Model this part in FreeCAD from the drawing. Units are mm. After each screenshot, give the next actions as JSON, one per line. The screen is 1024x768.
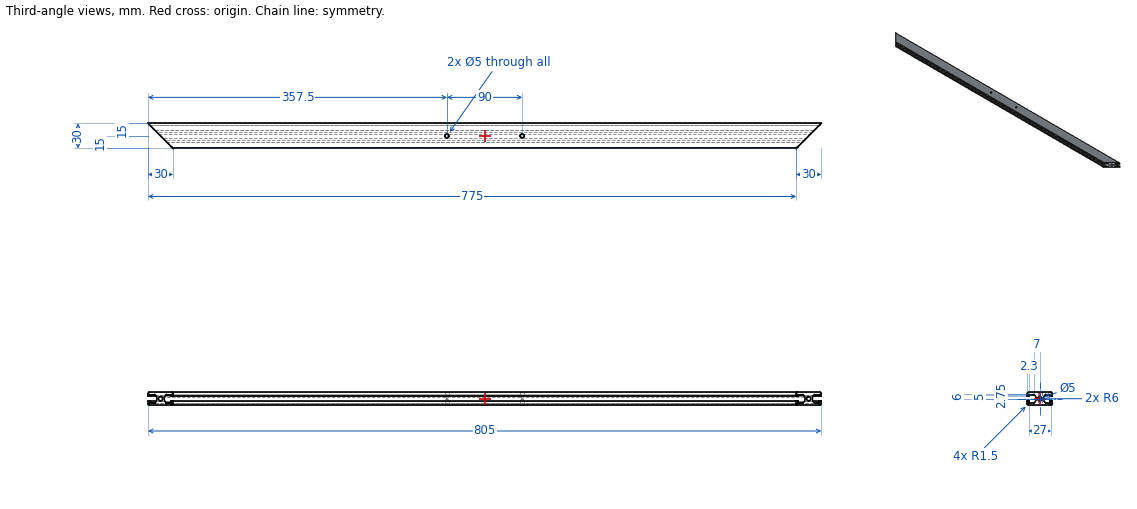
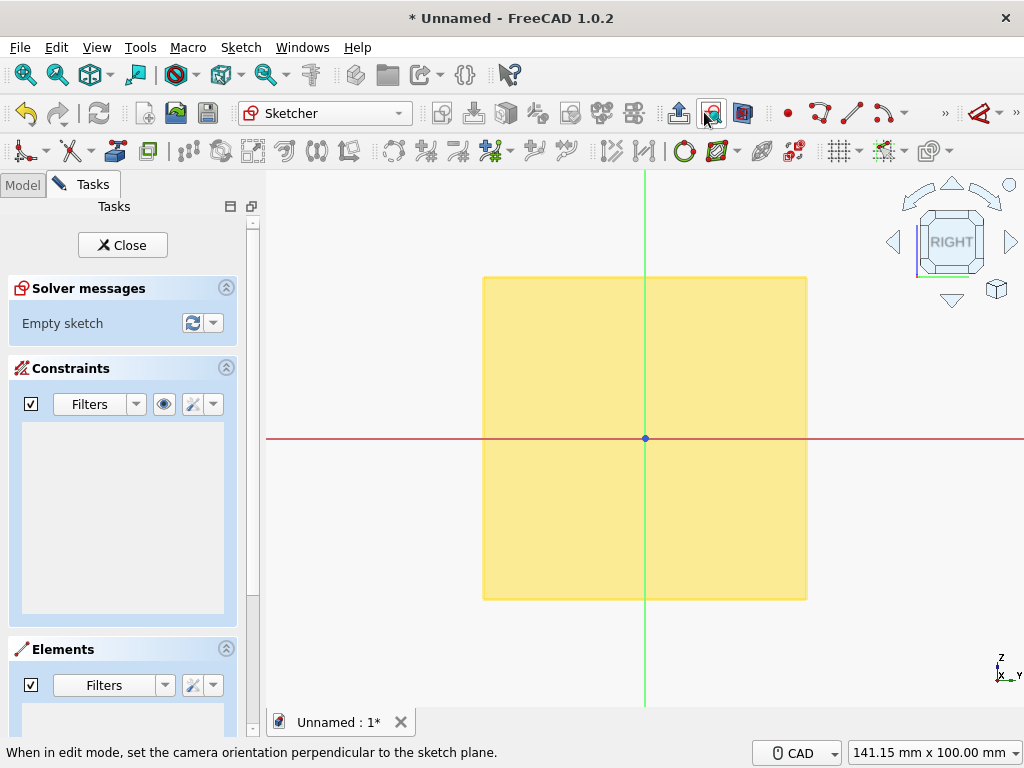
{"action": "scroll", "coordinate": [685, 439], "scroll_direction": "up", "scroll_amount": 5}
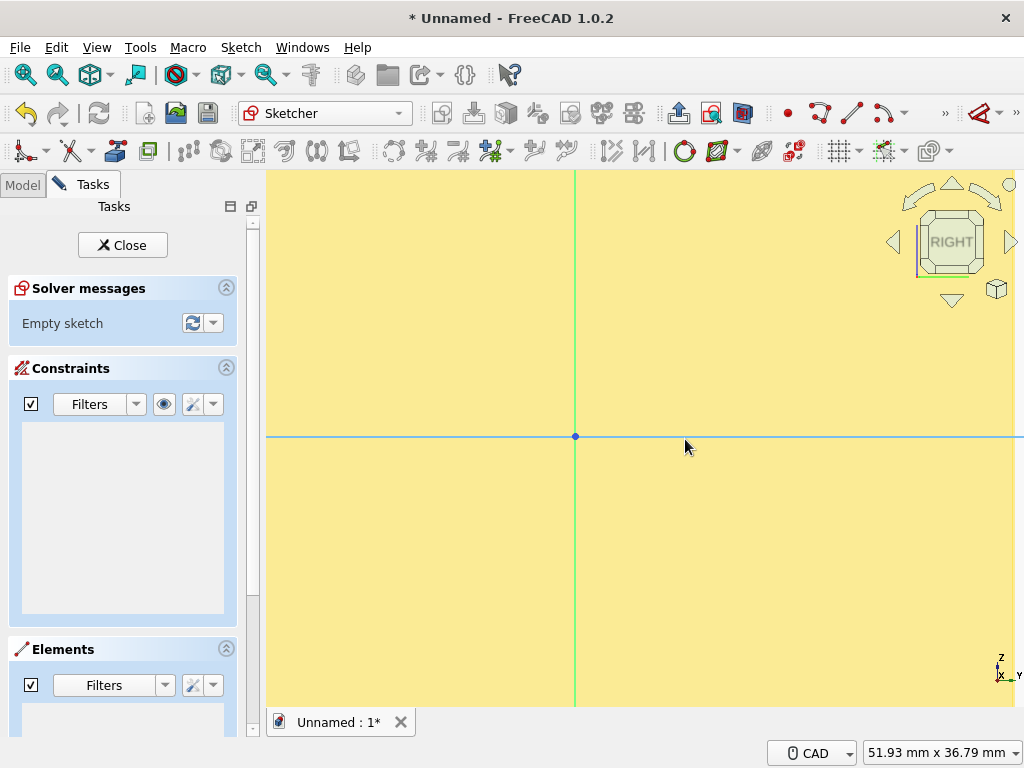
{"action": "left_click", "coordinate": [820, 114]}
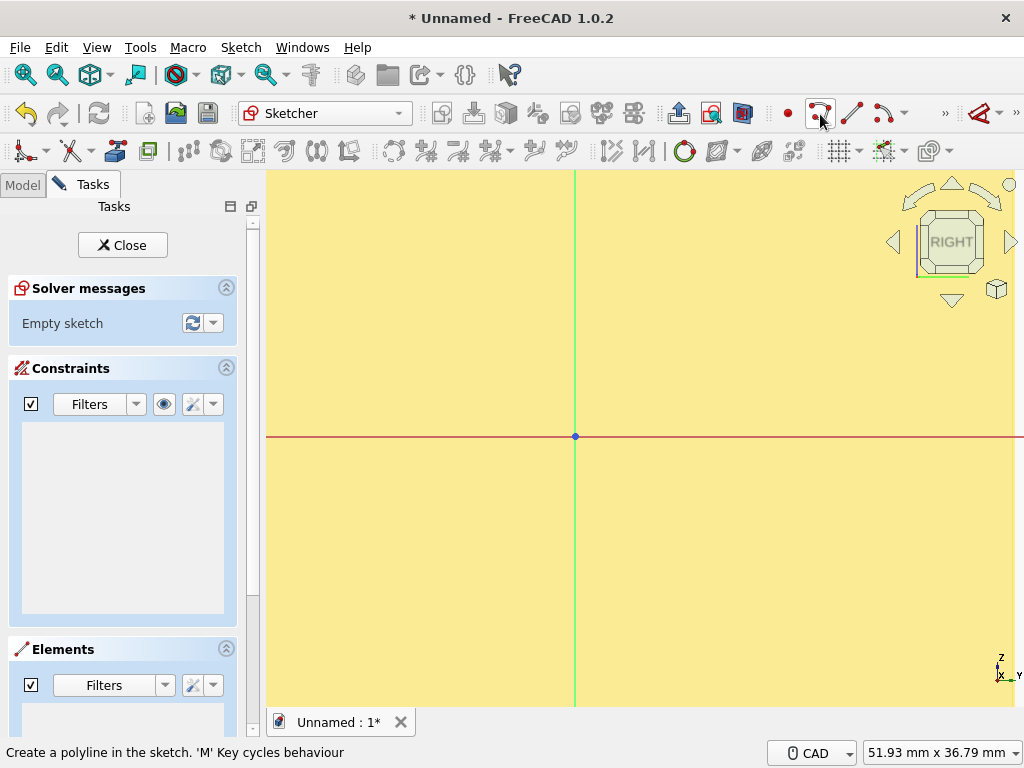
{"action": "left_click", "coordinate": [356, 349]}
{"action": "left_click", "coordinate": [356, 389]}
{"action": "left_click", "coordinate": [390, 389]}
{"action": "left_click", "coordinate": [390, 364]}
{"action": "left_click", "coordinate": [473, 364]}
{"action": "right_click", "coordinate": [473, 364]}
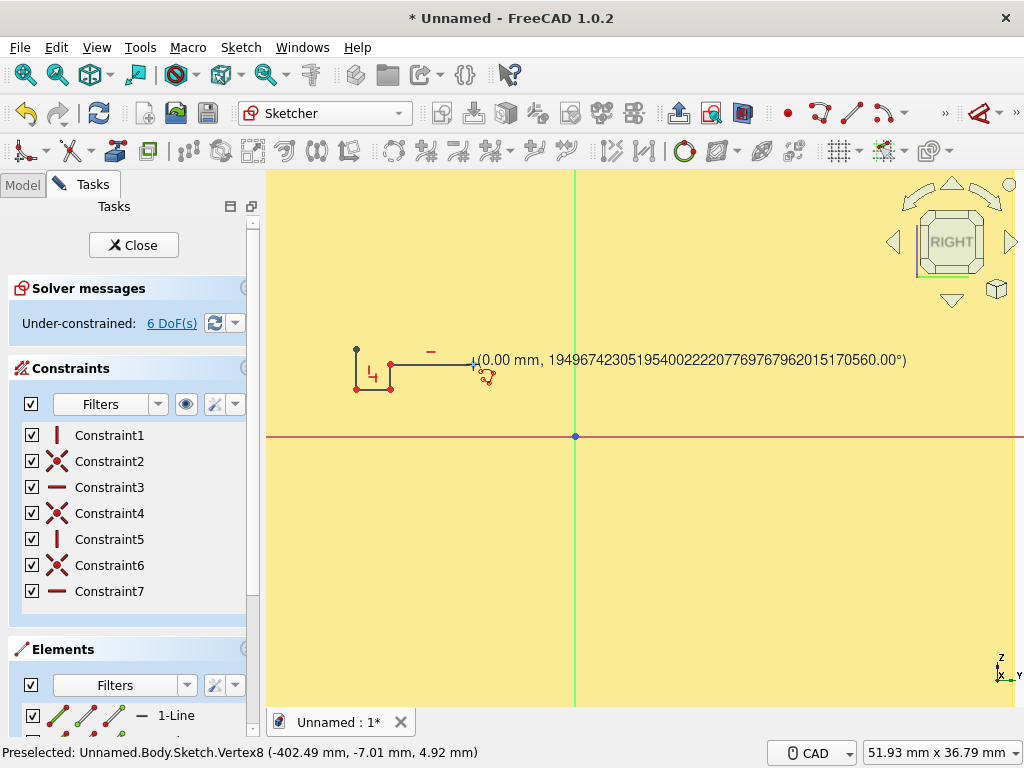
{"action": "left_click", "coordinate": [473, 510]}
{"action": "left_click", "coordinate": [390, 510]}
{"action": "left_click", "coordinate": [390, 484]}
{"action": "left_click", "coordinate": [356, 484]}
{"action": "left_click", "coordinate": [356, 524]}
{"action": "right_click", "coordinate": [356, 524]}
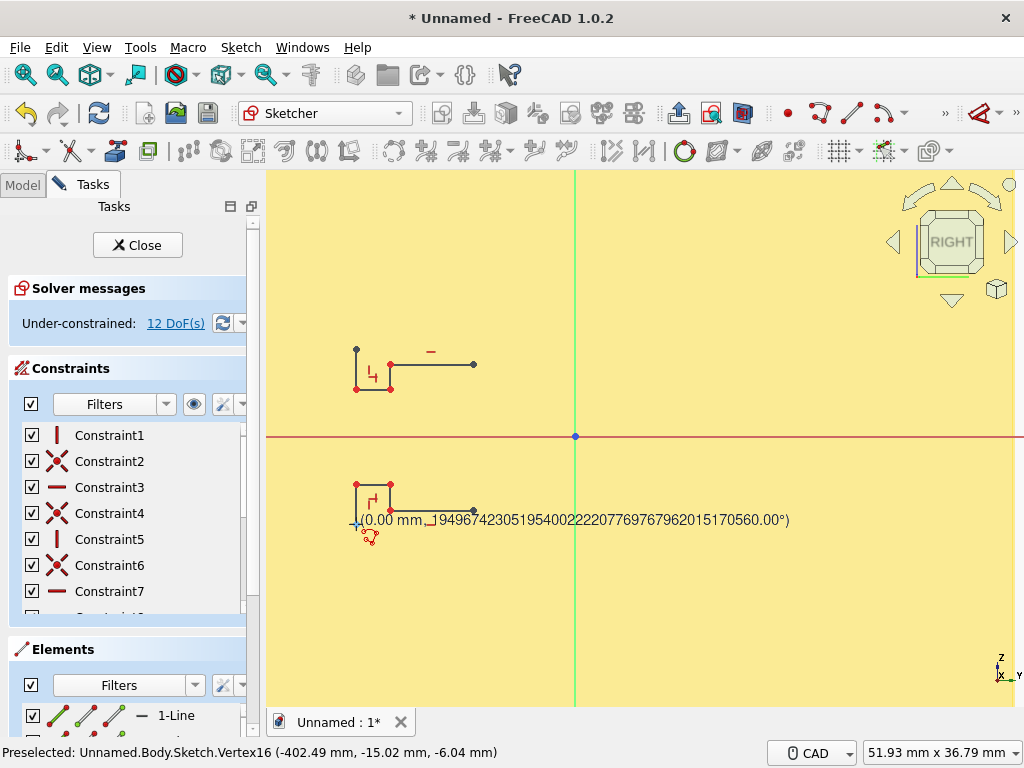
{"action": "left_click", "coordinate": [852, 114]}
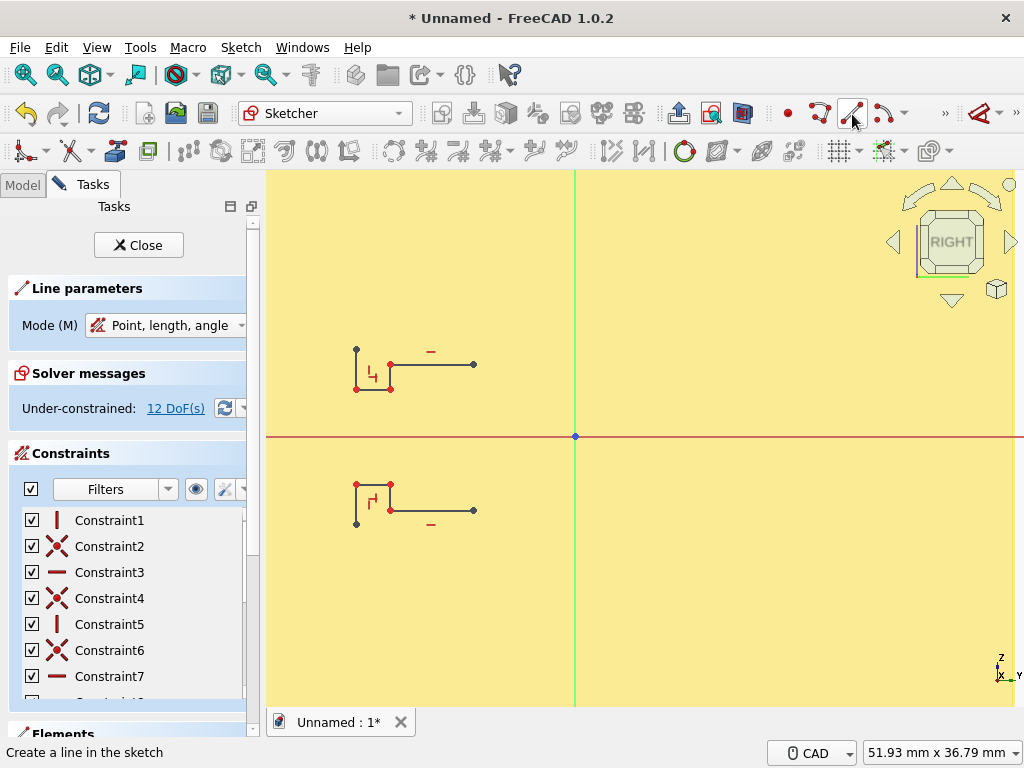
{"action": "left_click", "coordinate": [378, 546]}
{"action": "left_click", "coordinate": [772, 546]}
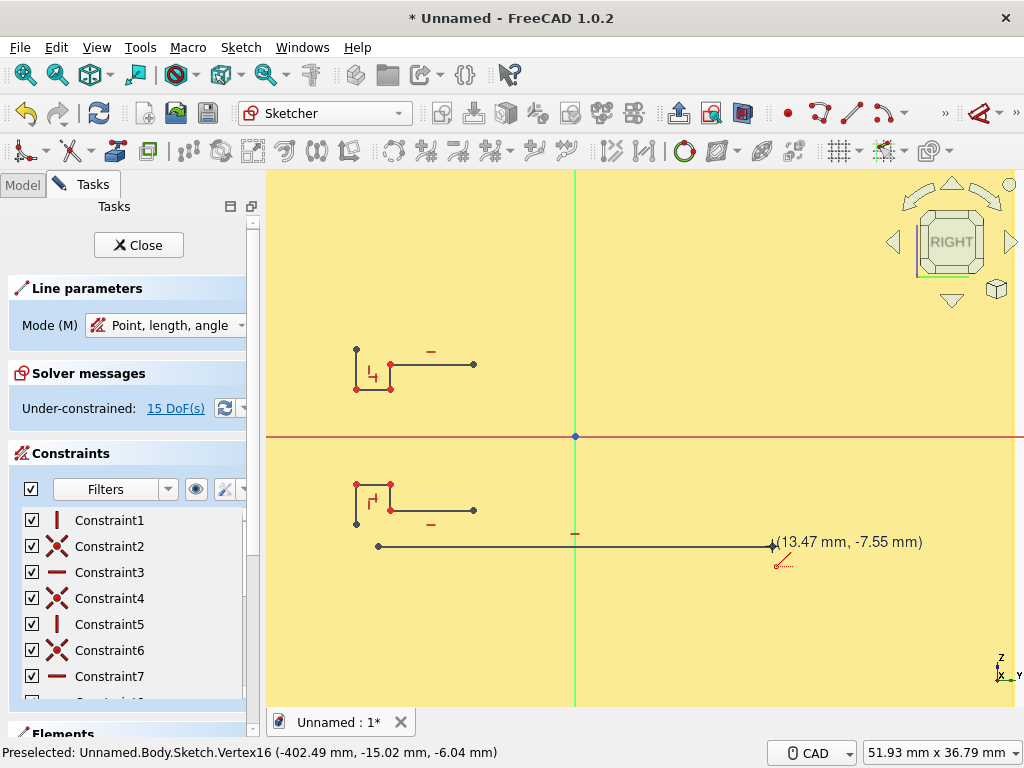
{"action": "left_click", "coordinate": [820, 114]}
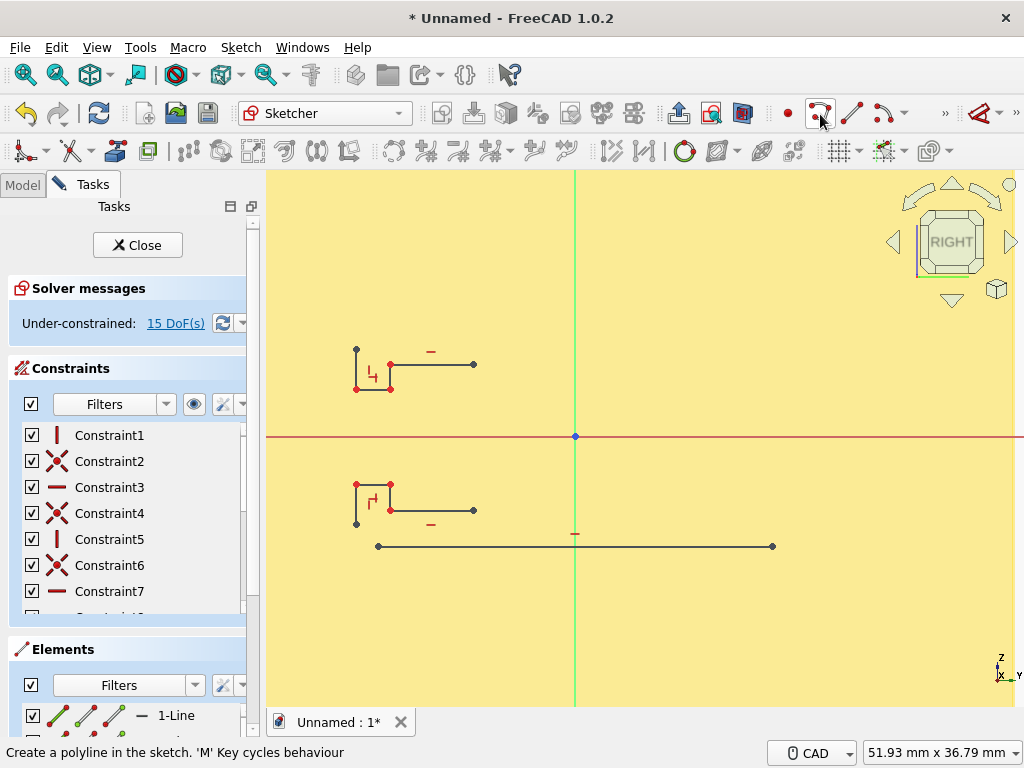
{"action": "left_click", "coordinate": [794, 524]}
{"action": "left_click", "coordinate": [794, 484]}
{"action": "left_click", "coordinate": [761, 484]}
{"action": "left_click", "coordinate": [761, 510]}
{"action": "left_click", "coordinate": [677, 510]}
{"action": "right_click", "coordinate": [677, 510]}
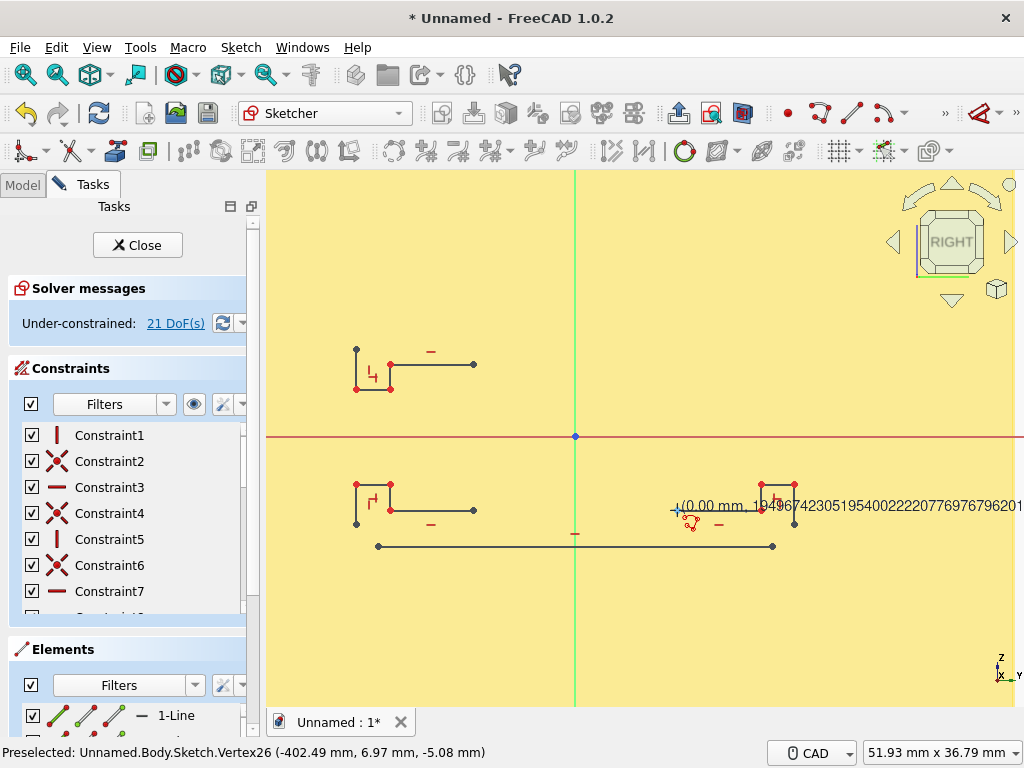
{"action": "left_click", "coordinate": [677, 364]}
{"action": "left_click", "coordinate": [761, 364]}
{"action": "left_click", "coordinate": [761, 389]}
{"action": "left_click", "coordinate": [794, 389]}
{"action": "left_click", "coordinate": [794, 349]}
{"action": "right_click", "coordinate": [794, 349]}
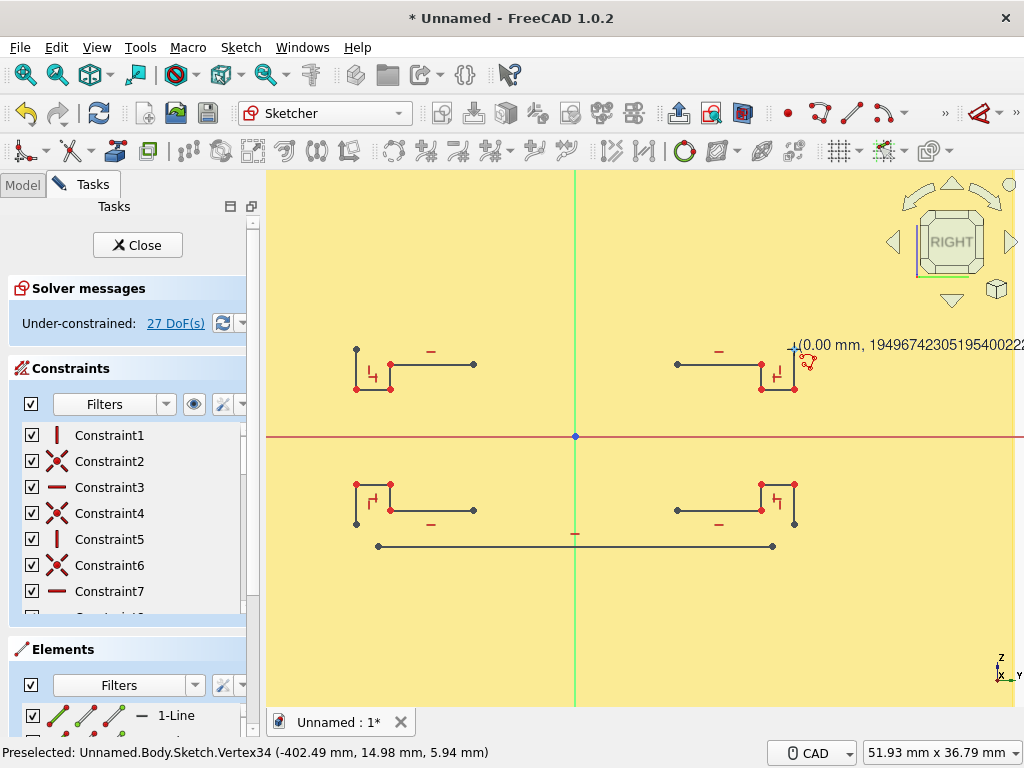
{"action": "left_click", "coordinate": [852, 114]}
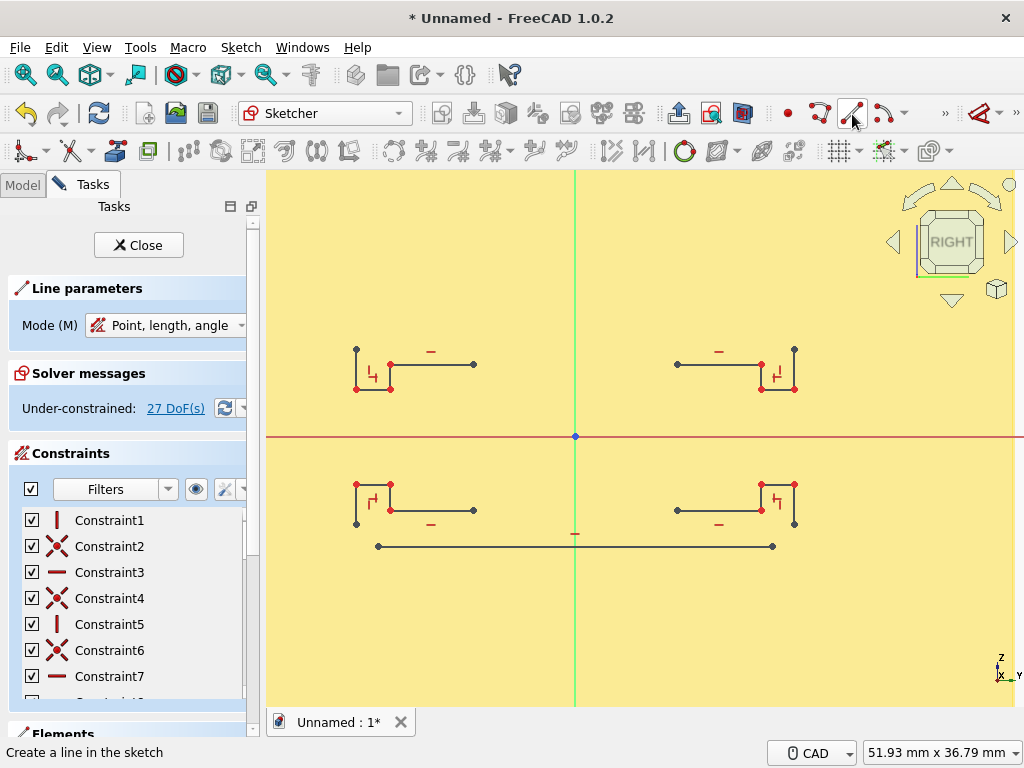
{"action": "left_click", "coordinate": [772, 327]}
{"action": "left_click", "coordinate": [378, 327]}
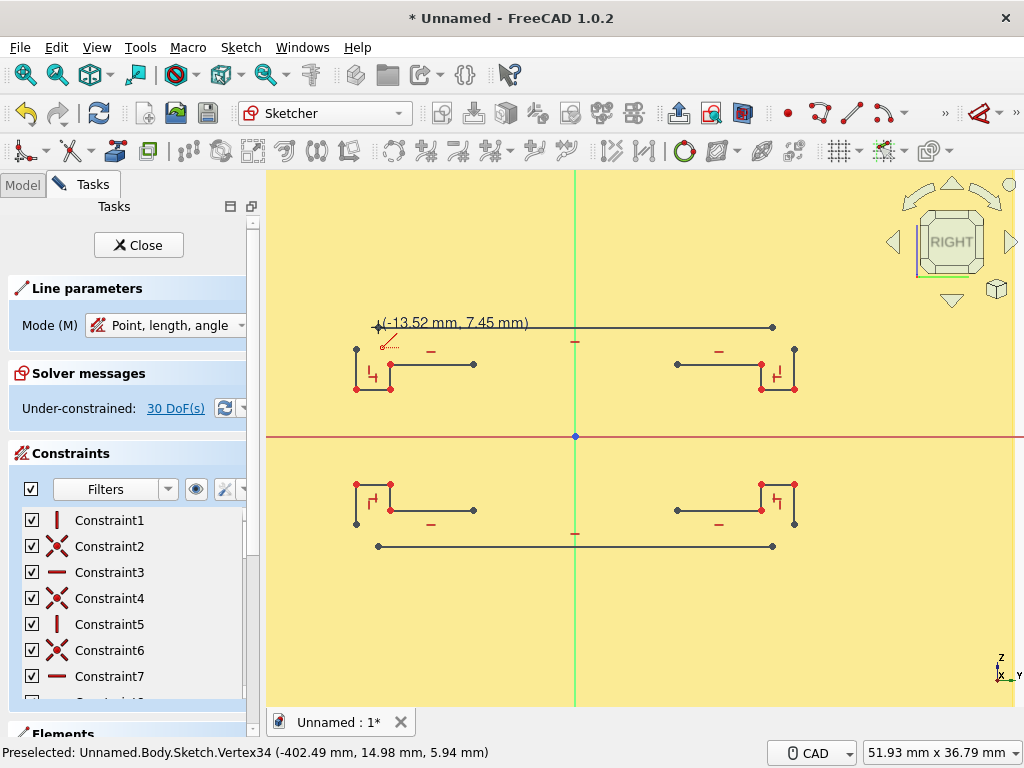
{"action": "left_click", "coordinate": [906, 114]}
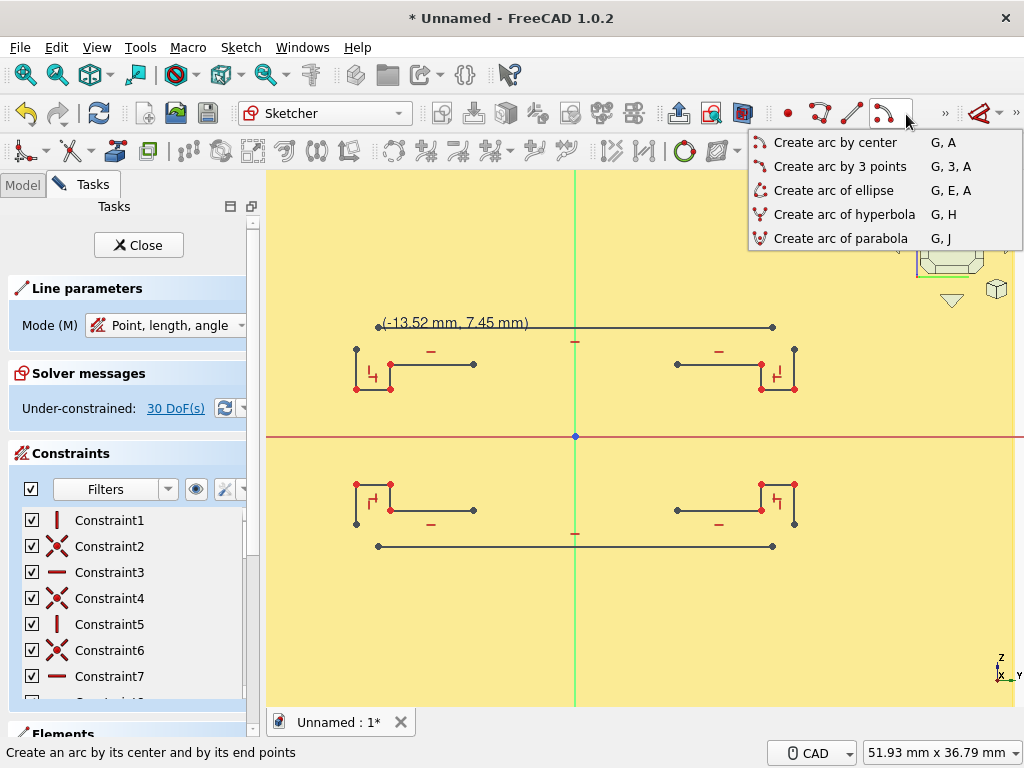
{"action": "left_click", "coordinate": [886, 166]}